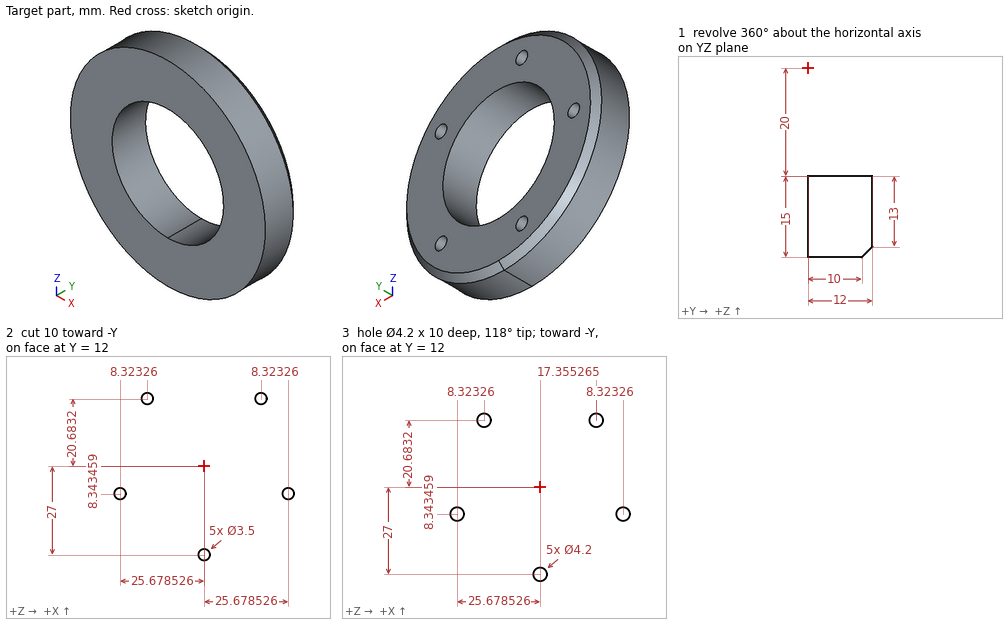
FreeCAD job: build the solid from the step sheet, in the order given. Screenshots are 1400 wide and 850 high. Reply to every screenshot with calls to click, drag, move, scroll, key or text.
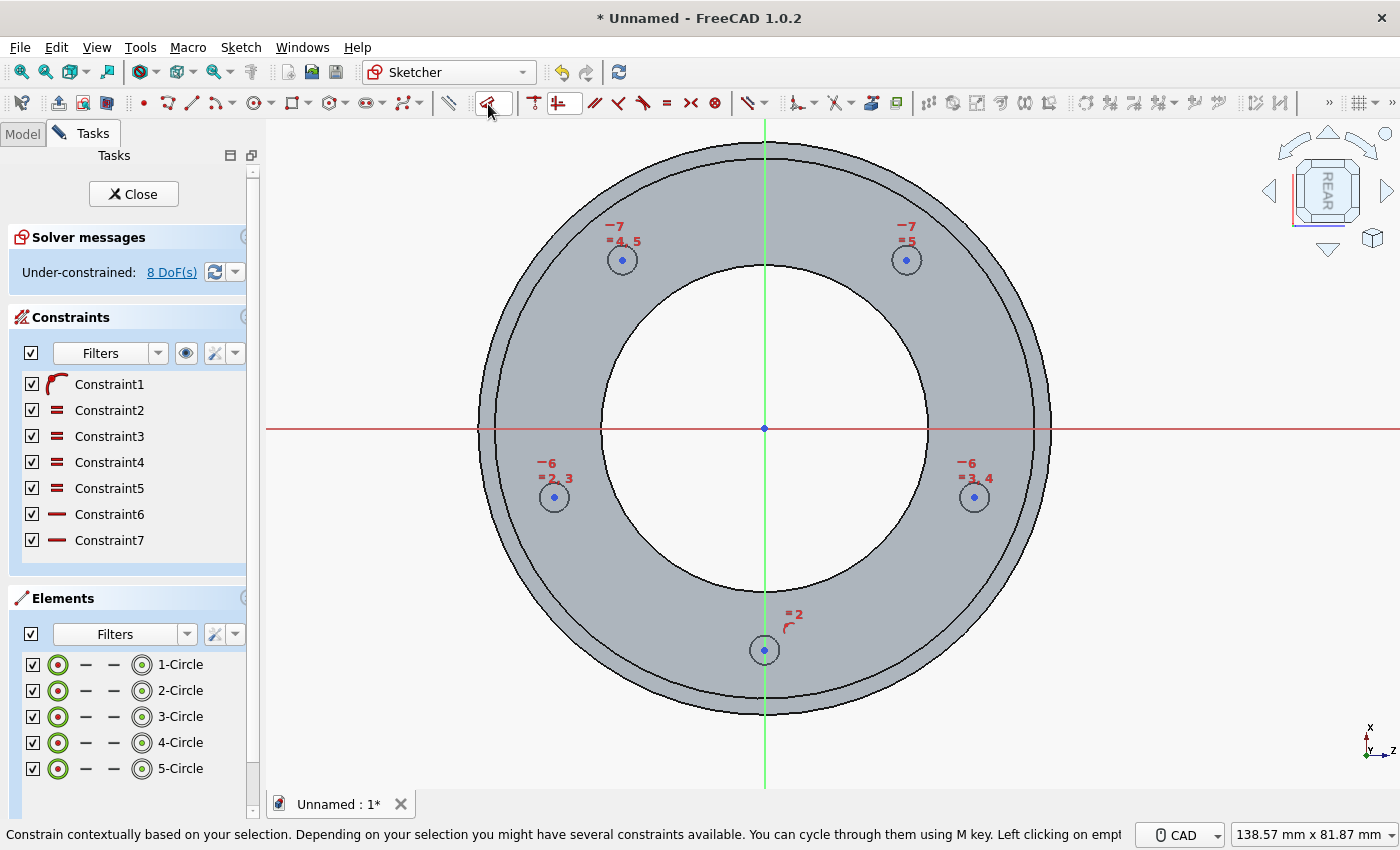
scroll(775, 640, up, 2)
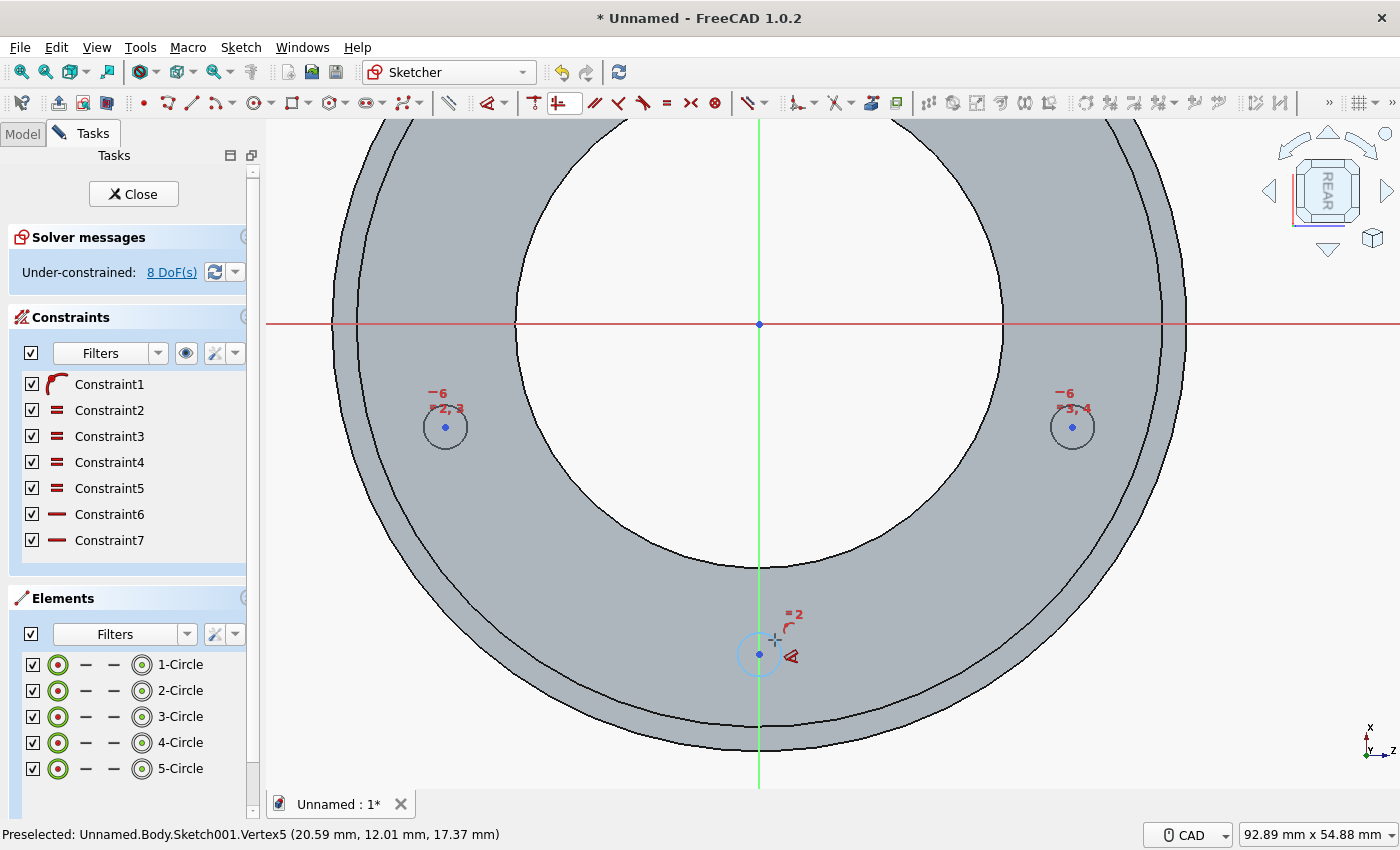
click(775, 639)
click(798, 616)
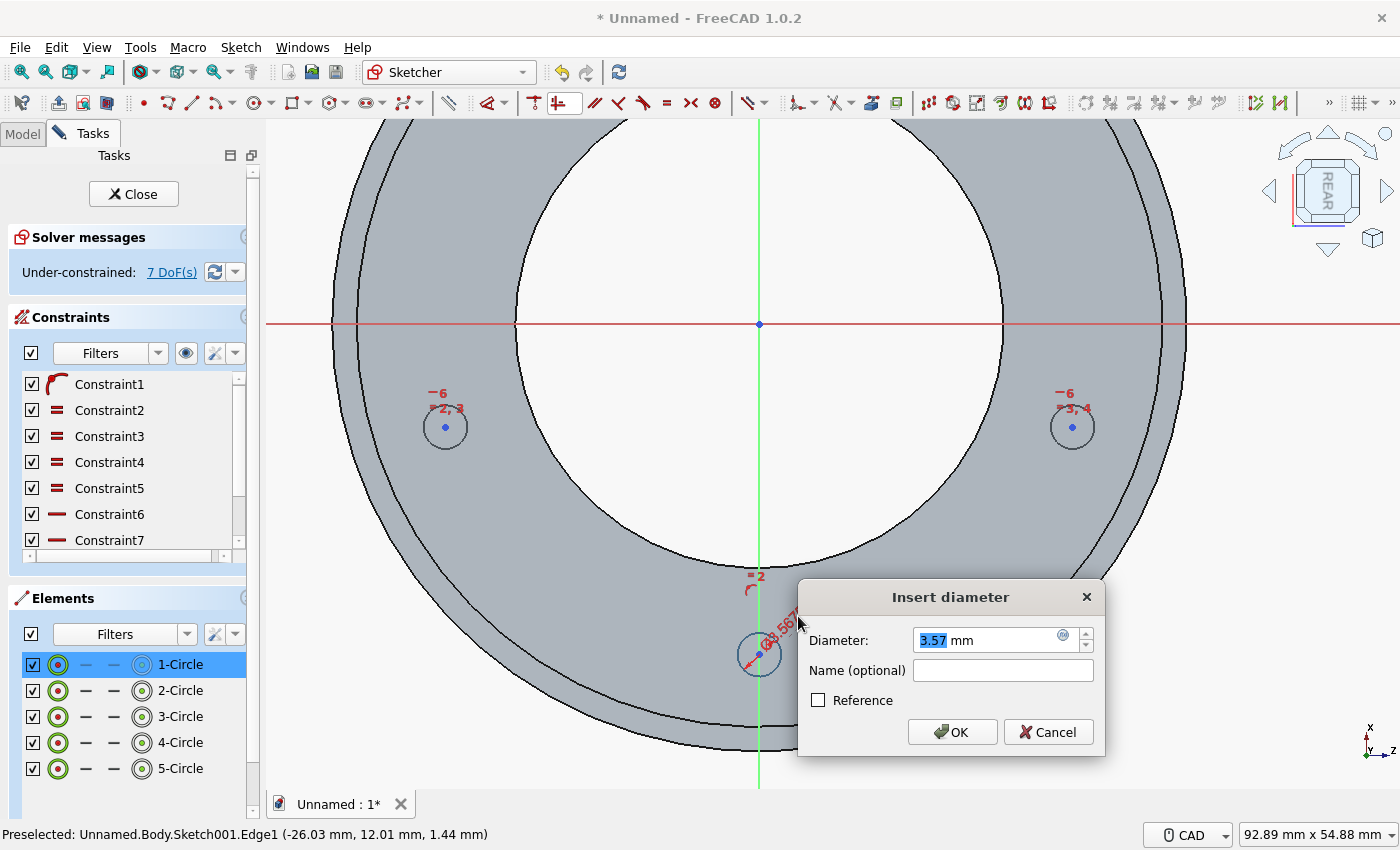
text(3.5)
key(Return)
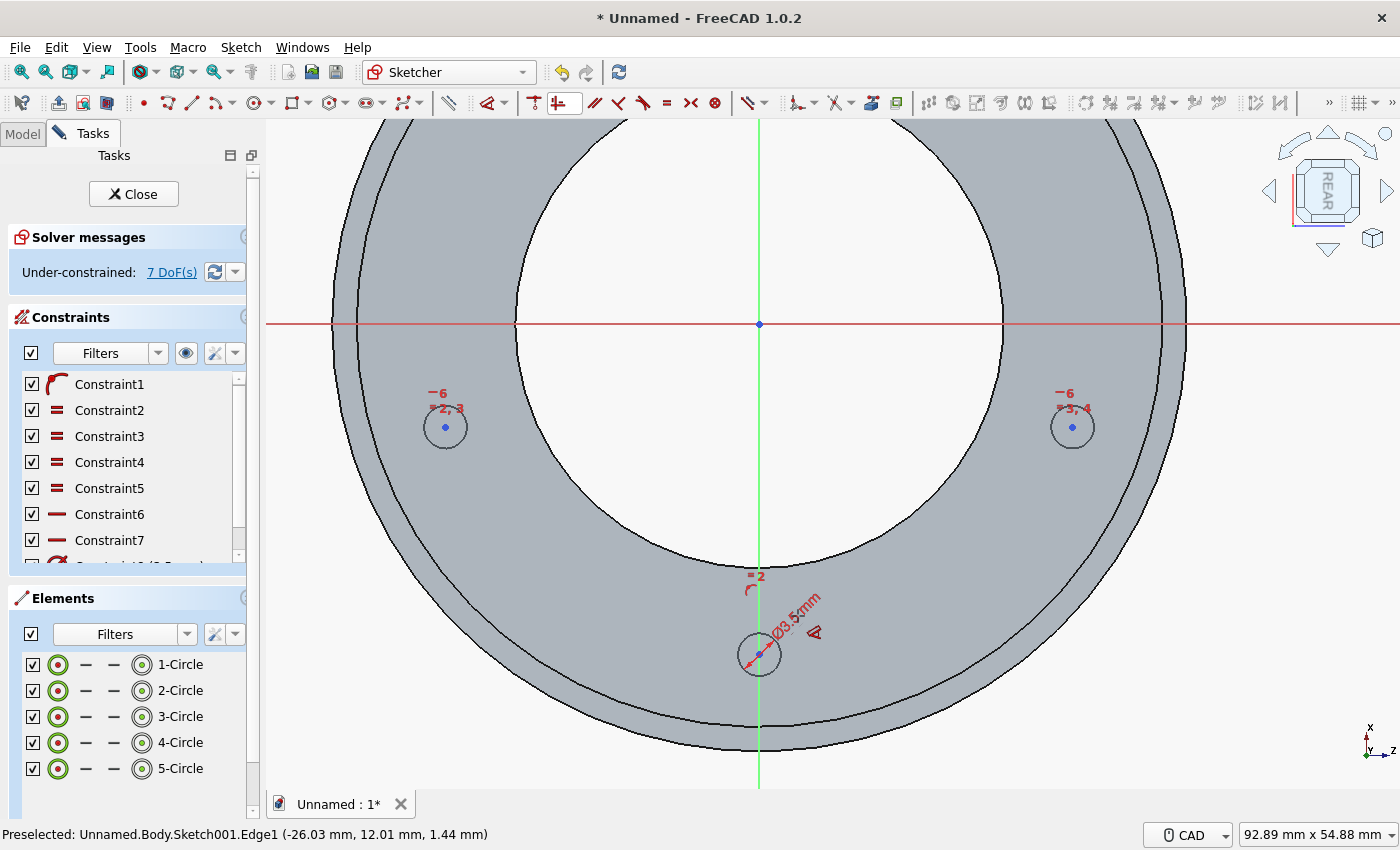
click(759, 655)
click(793, 489)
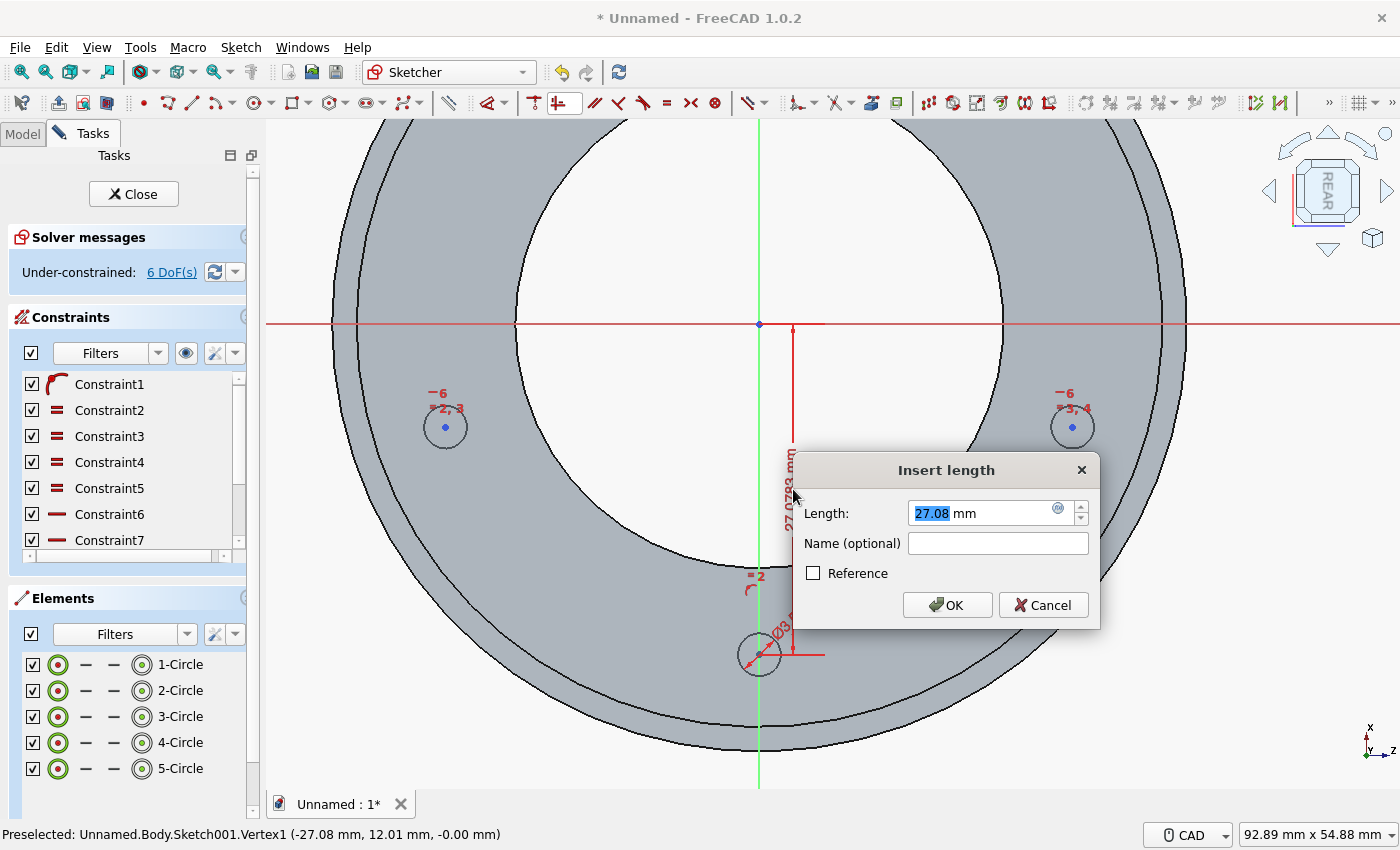
text(27)
key(Return)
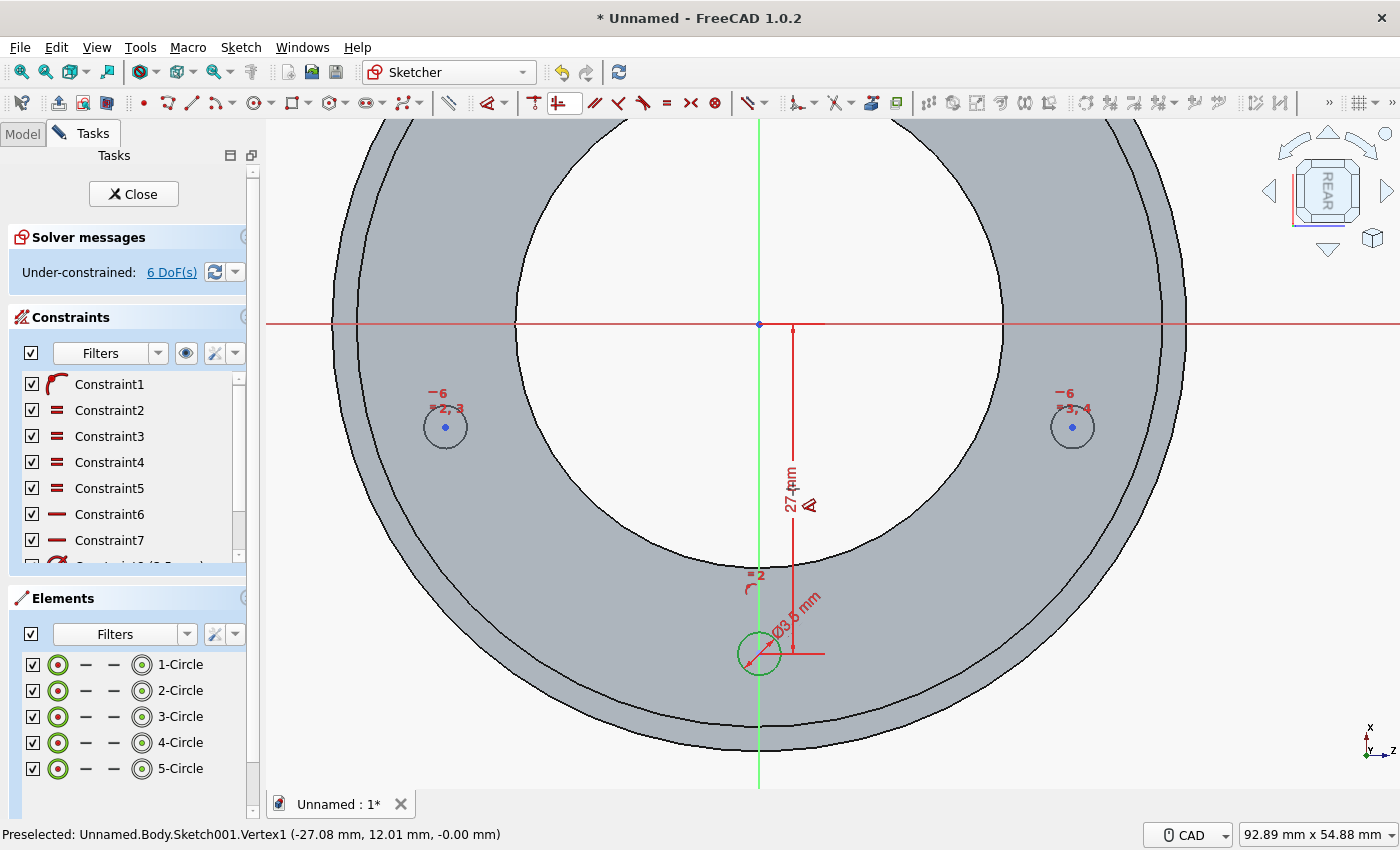
scroll(775, 640, down, 2)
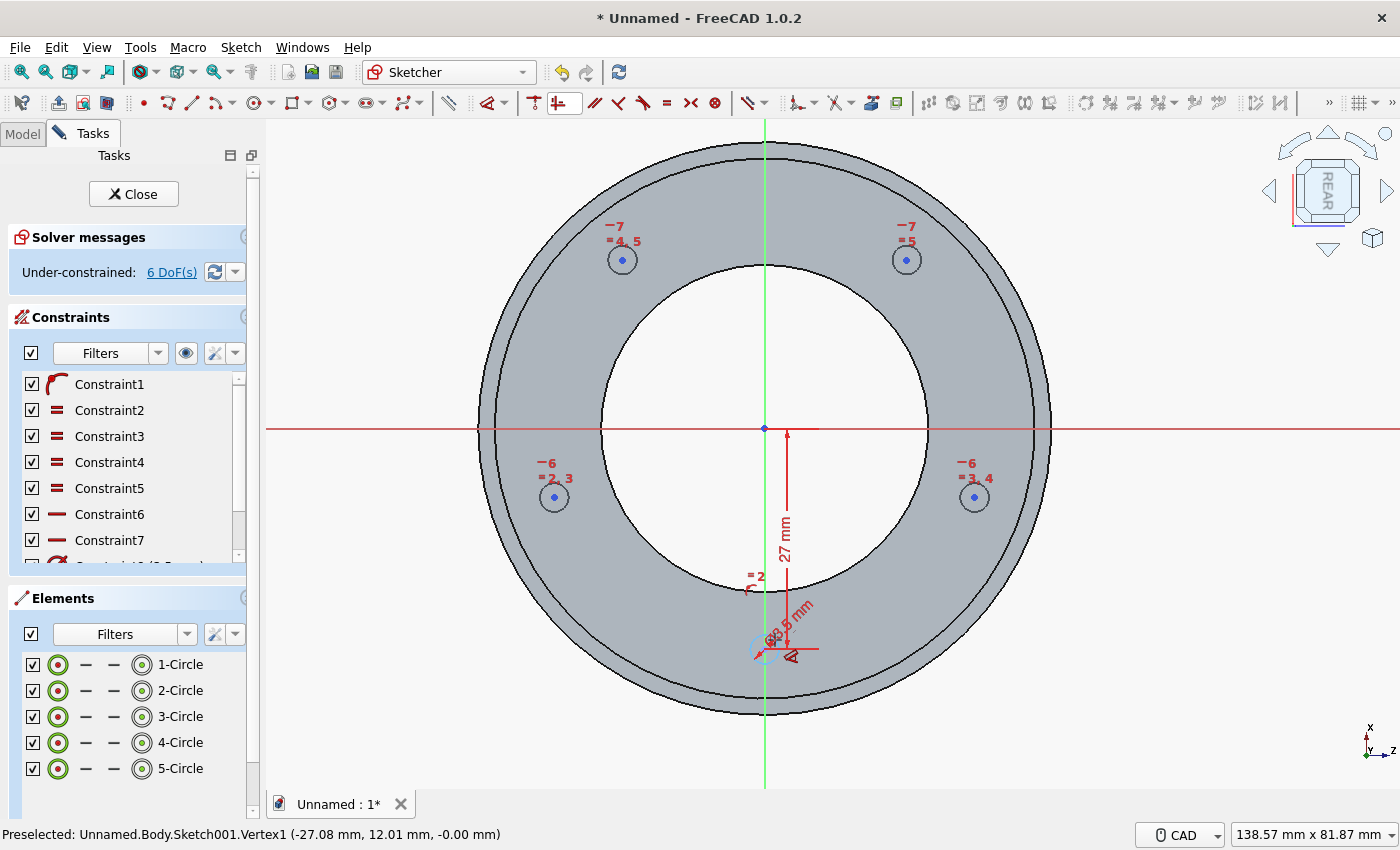
click(623, 260)
click(589, 344)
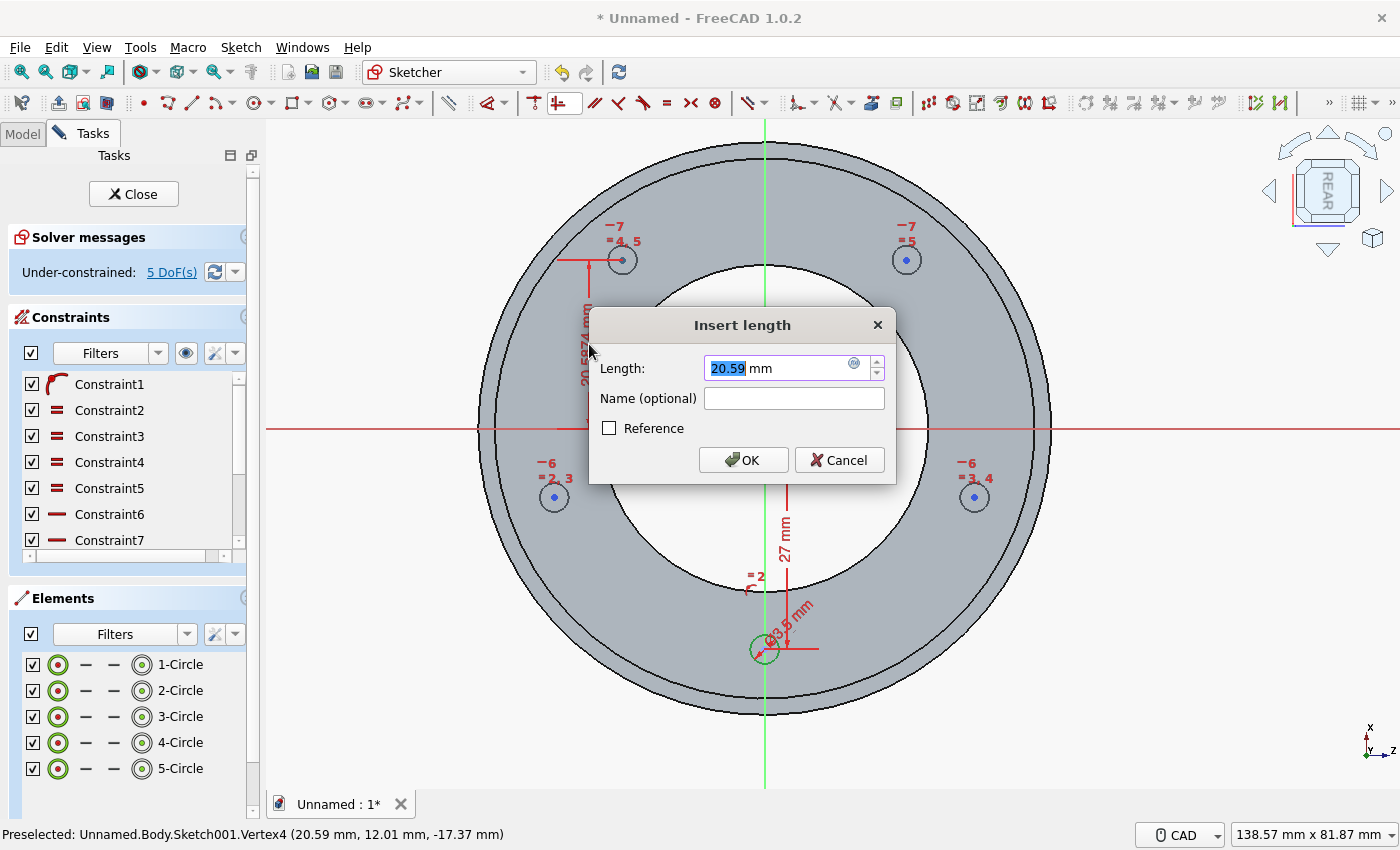
text(20.6832)
key(Return)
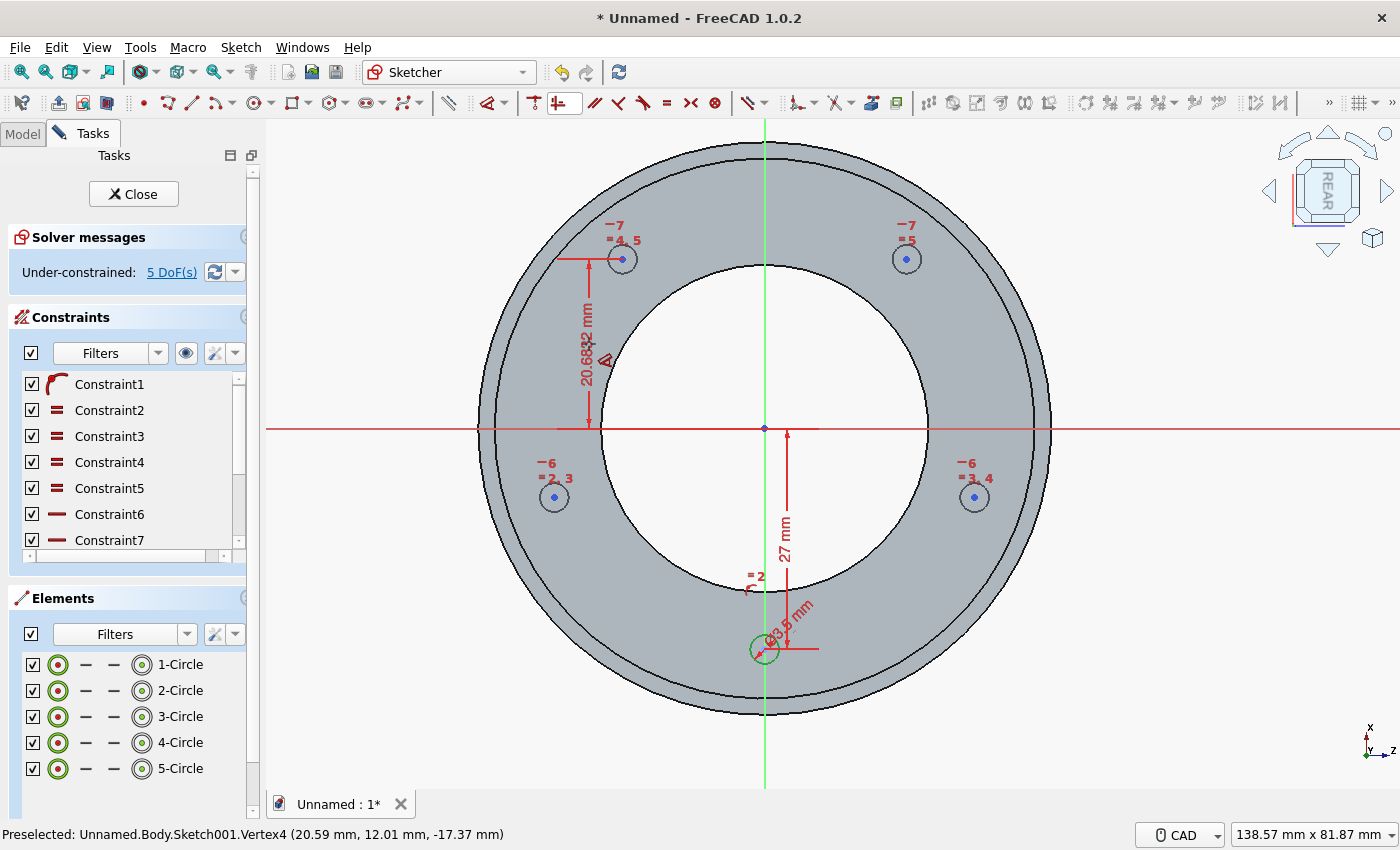
click(554, 498)
click(520, 463)